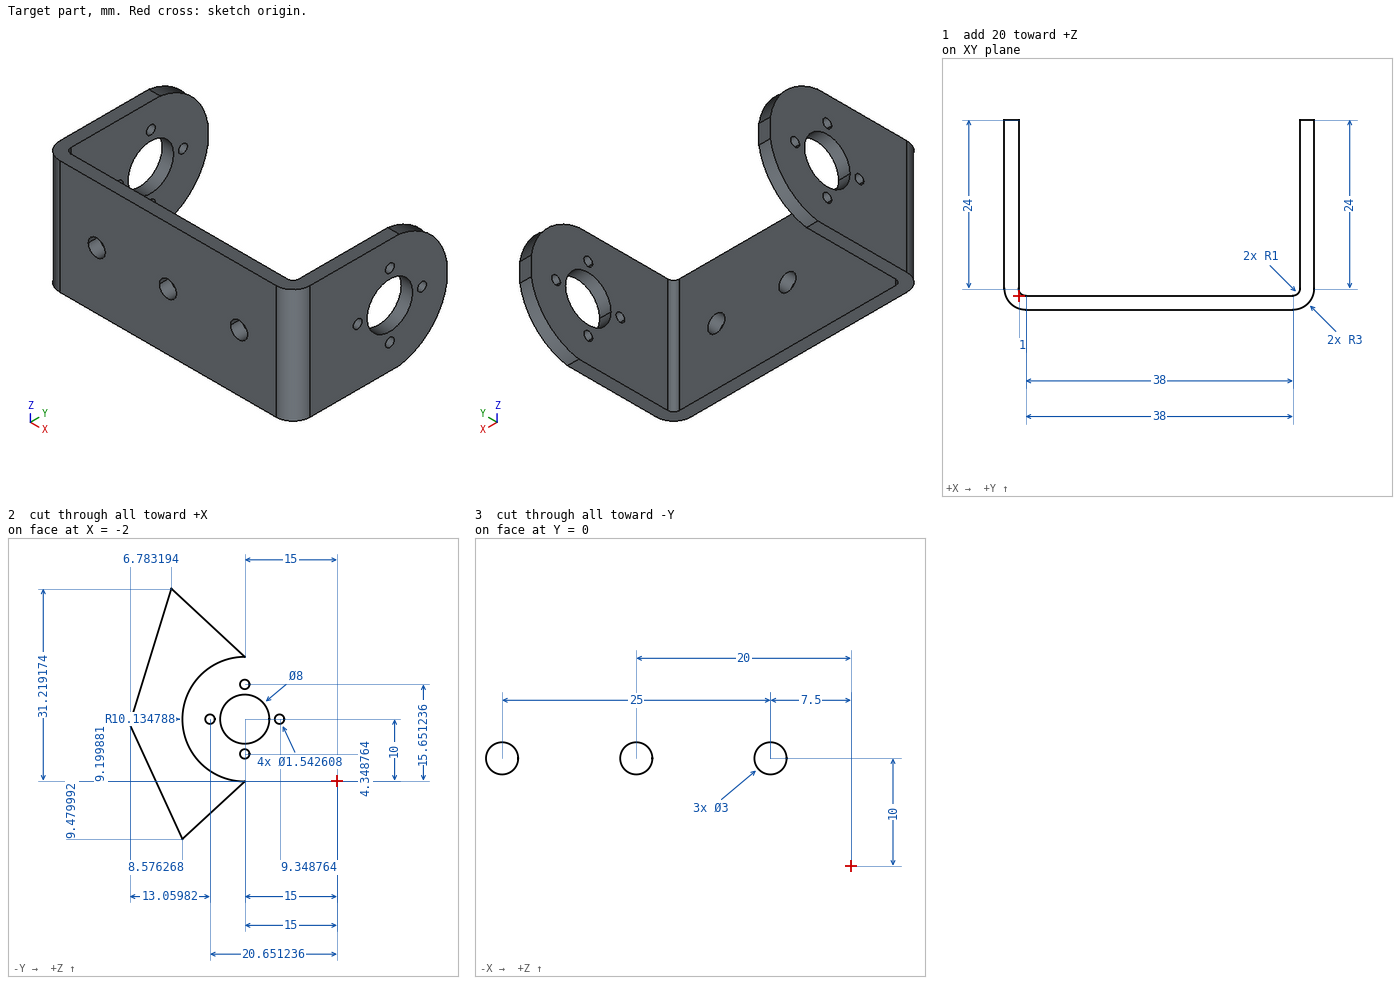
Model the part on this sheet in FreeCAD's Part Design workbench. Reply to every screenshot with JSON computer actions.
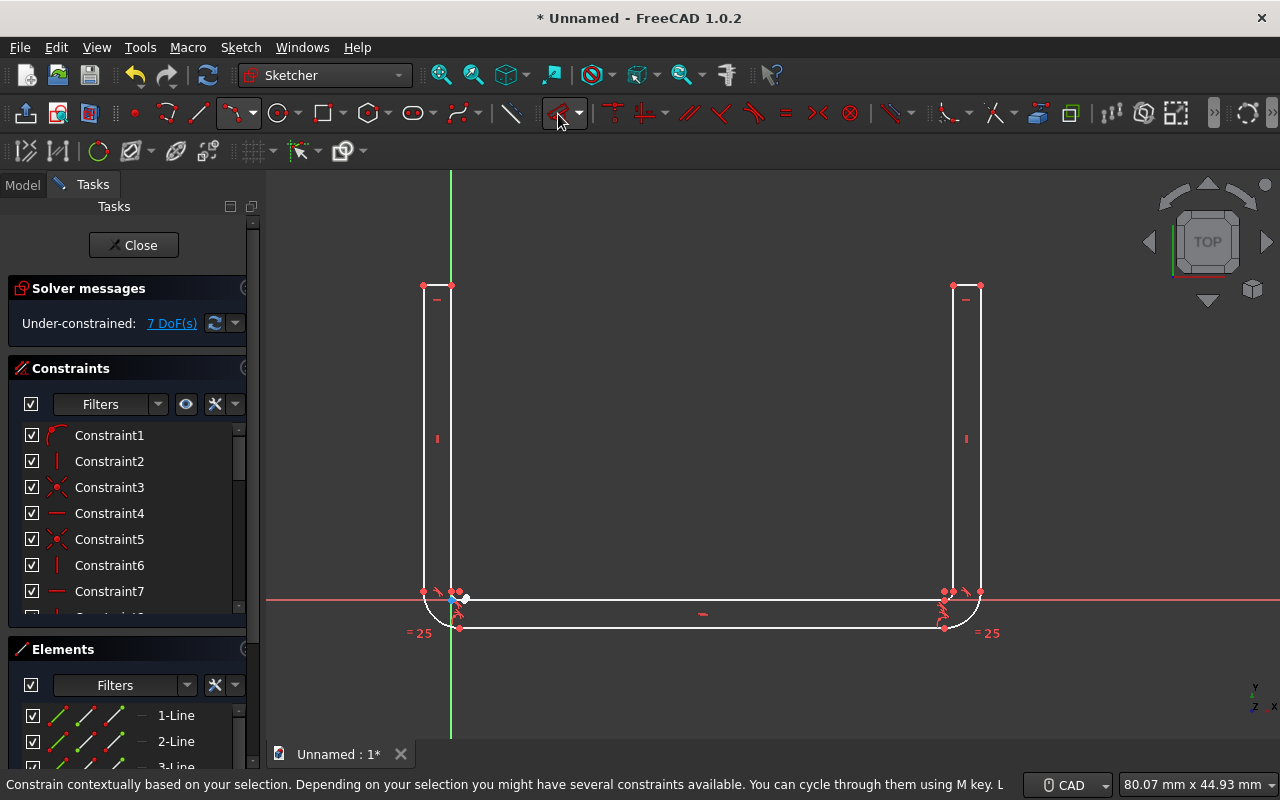
{"action": "left_click", "coordinate": [434, 617]}
{"action": "left_click", "coordinate": [411, 639]}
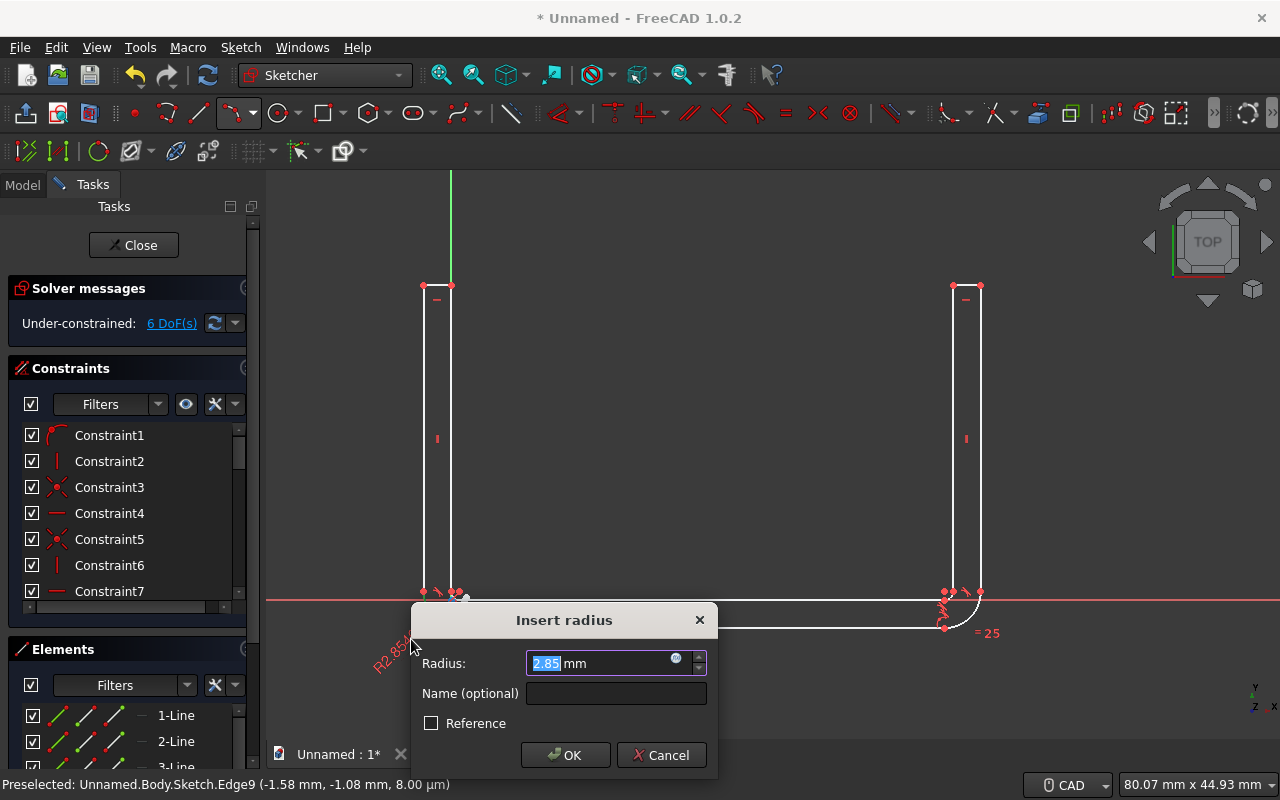
{"action": "type", "text": "3"}
{"action": "key", "text": "Return"}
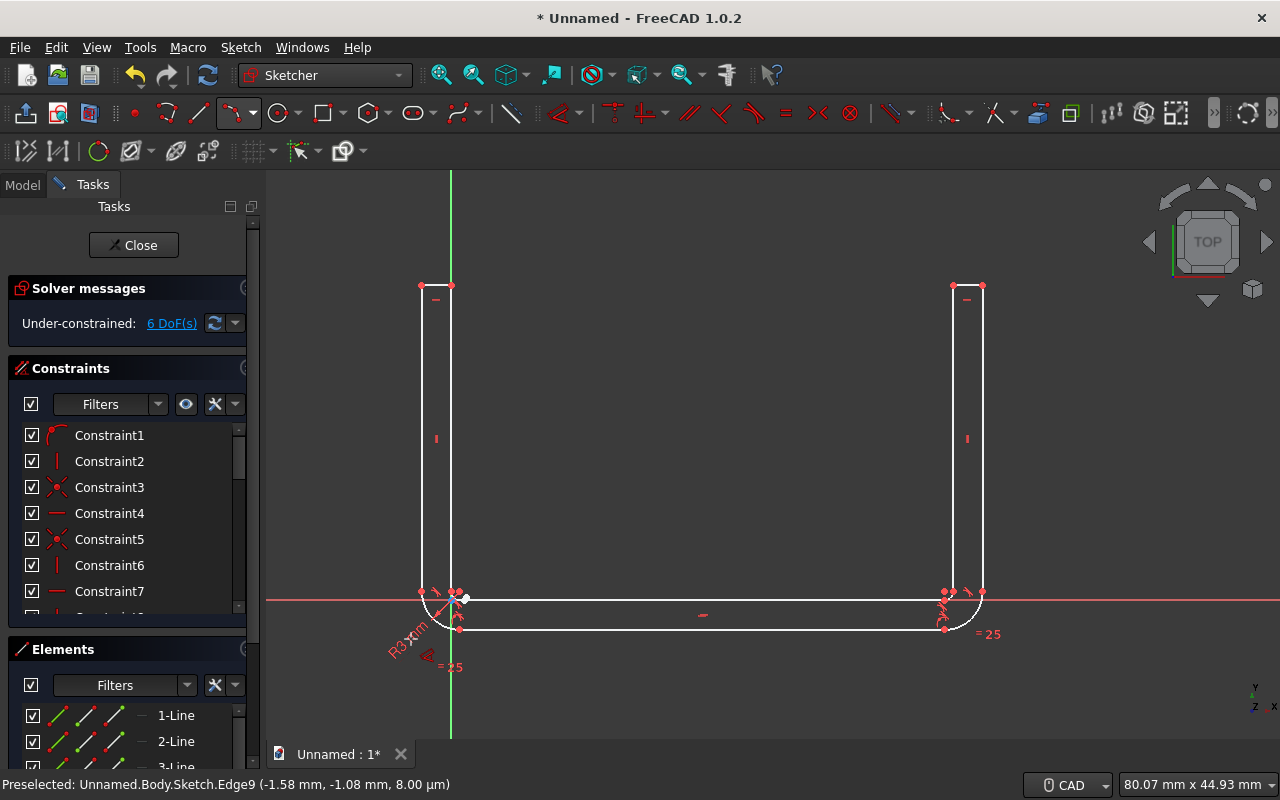
{"action": "scroll", "coordinate": [951, 598], "scroll_direction": "up", "scroll_amount": 6}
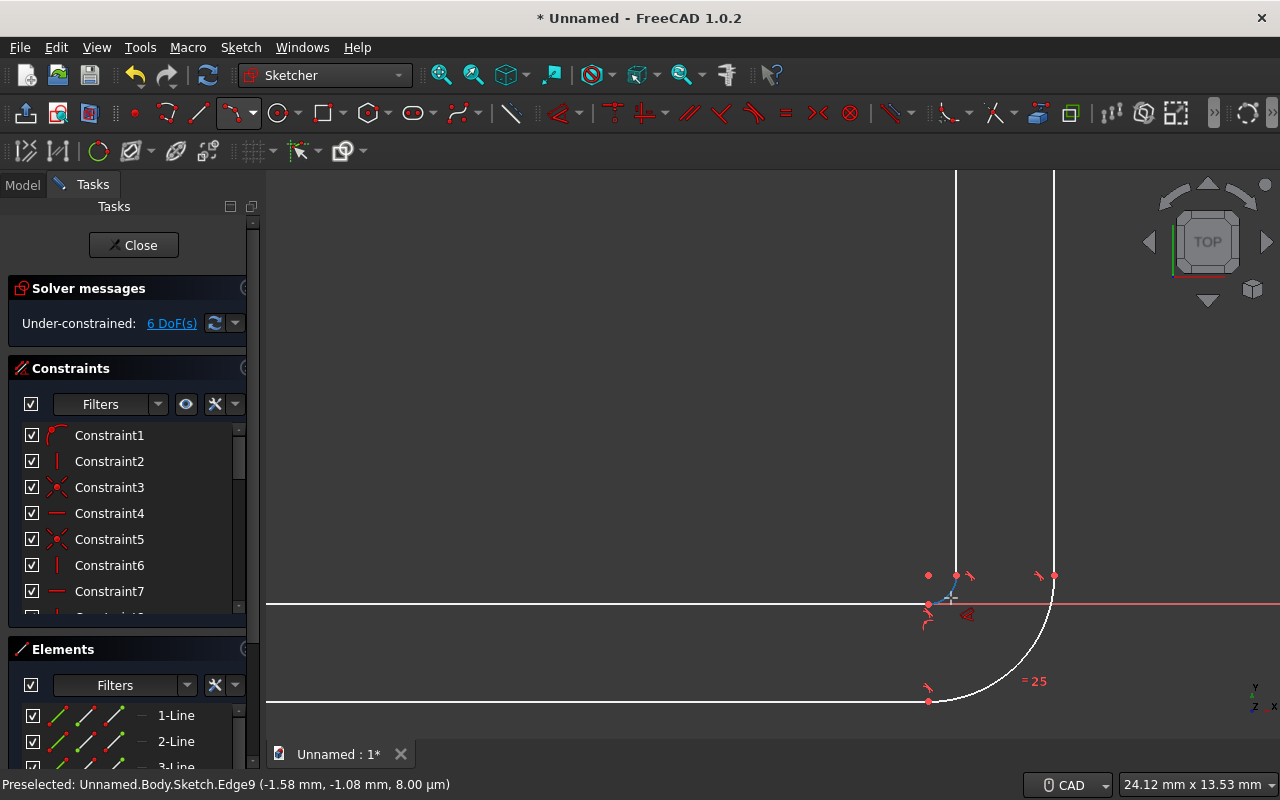
{"action": "left_click", "coordinate": [948, 596]}
{"action": "left_click", "coordinate": [971, 619]}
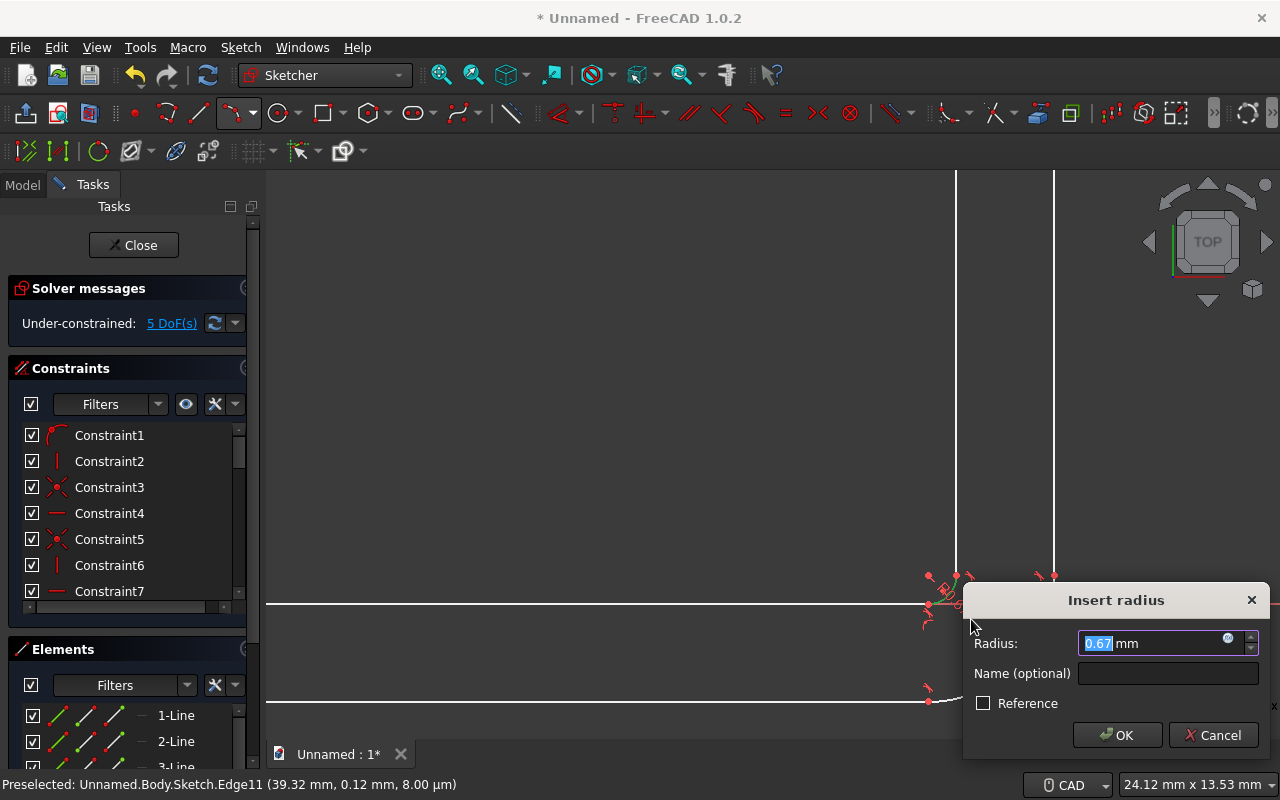
{"action": "type", "text": "1"}
{"action": "key", "text": "Return"}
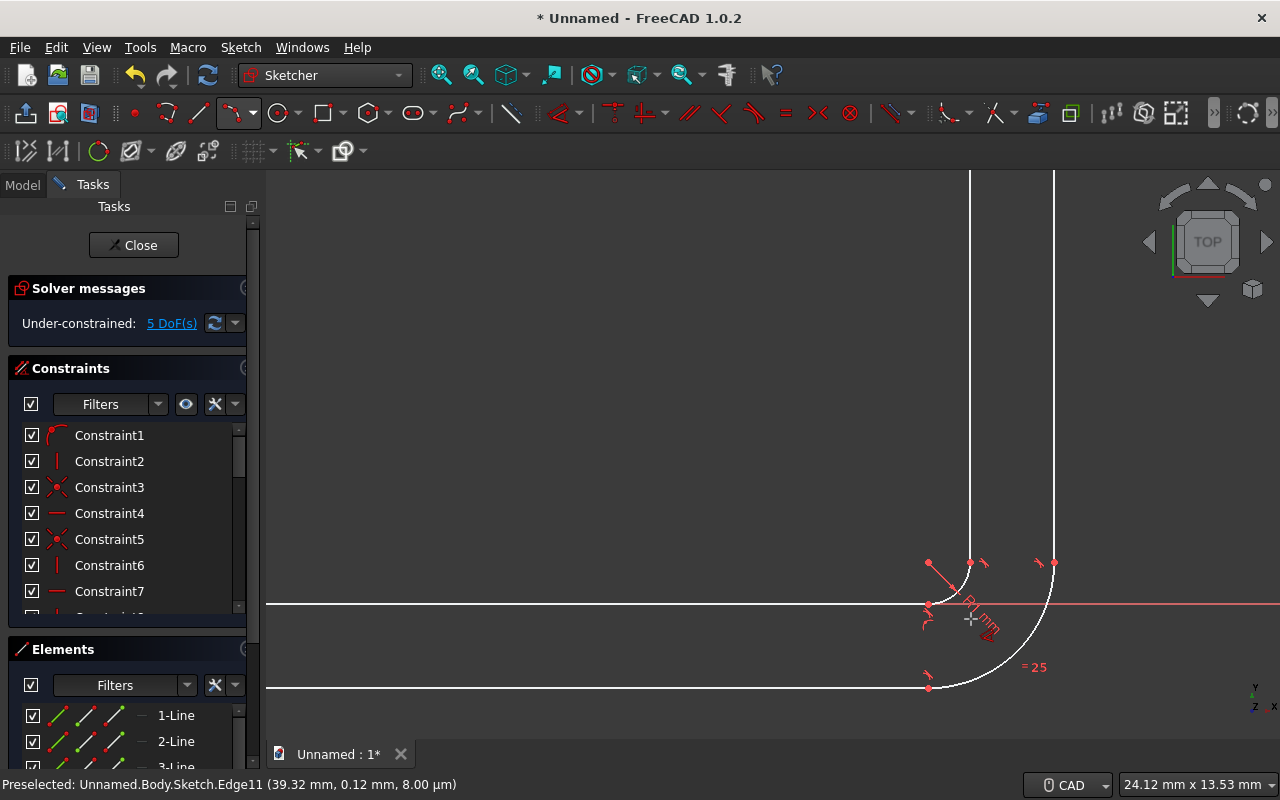
{"action": "scroll", "coordinate": [951, 598], "scroll_direction": "down", "scroll_amount": 6}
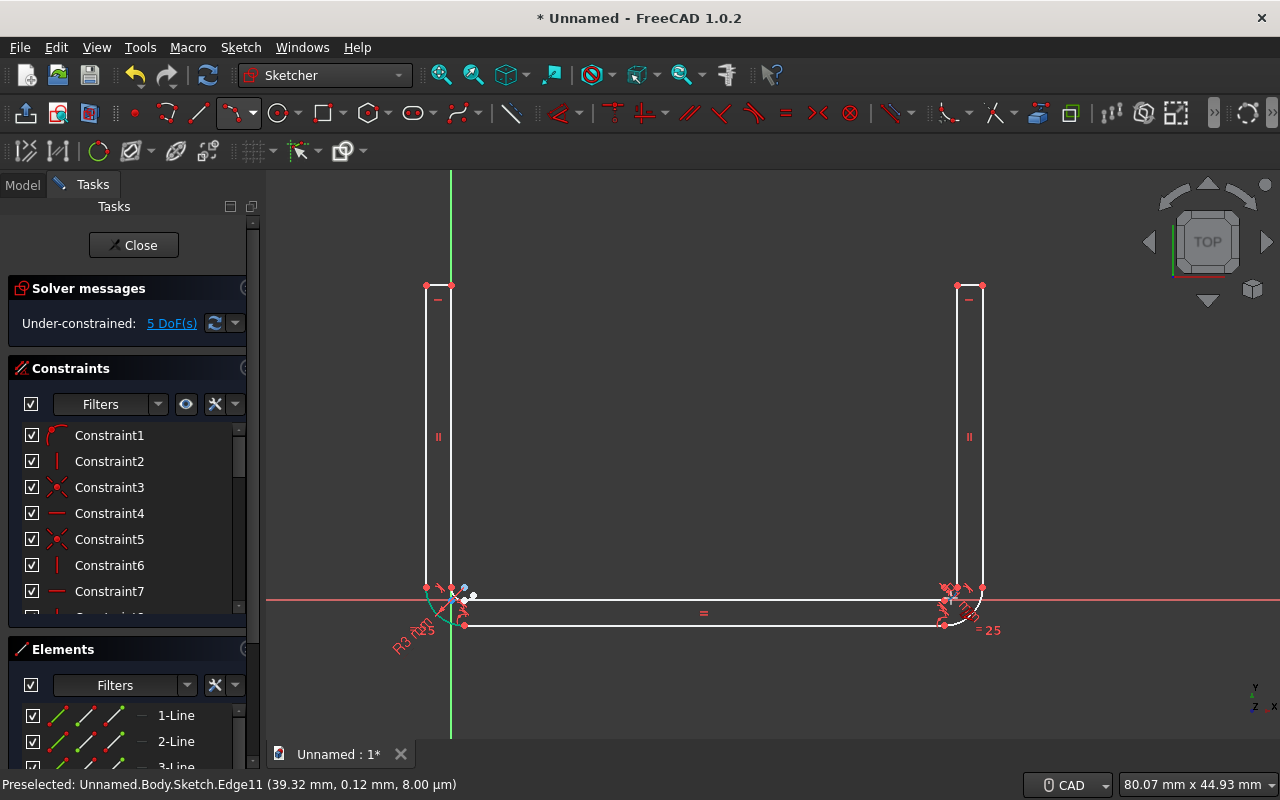
{"action": "left_click", "coordinate": [451, 497]}
{"action": "left_click", "coordinate": [485, 436]}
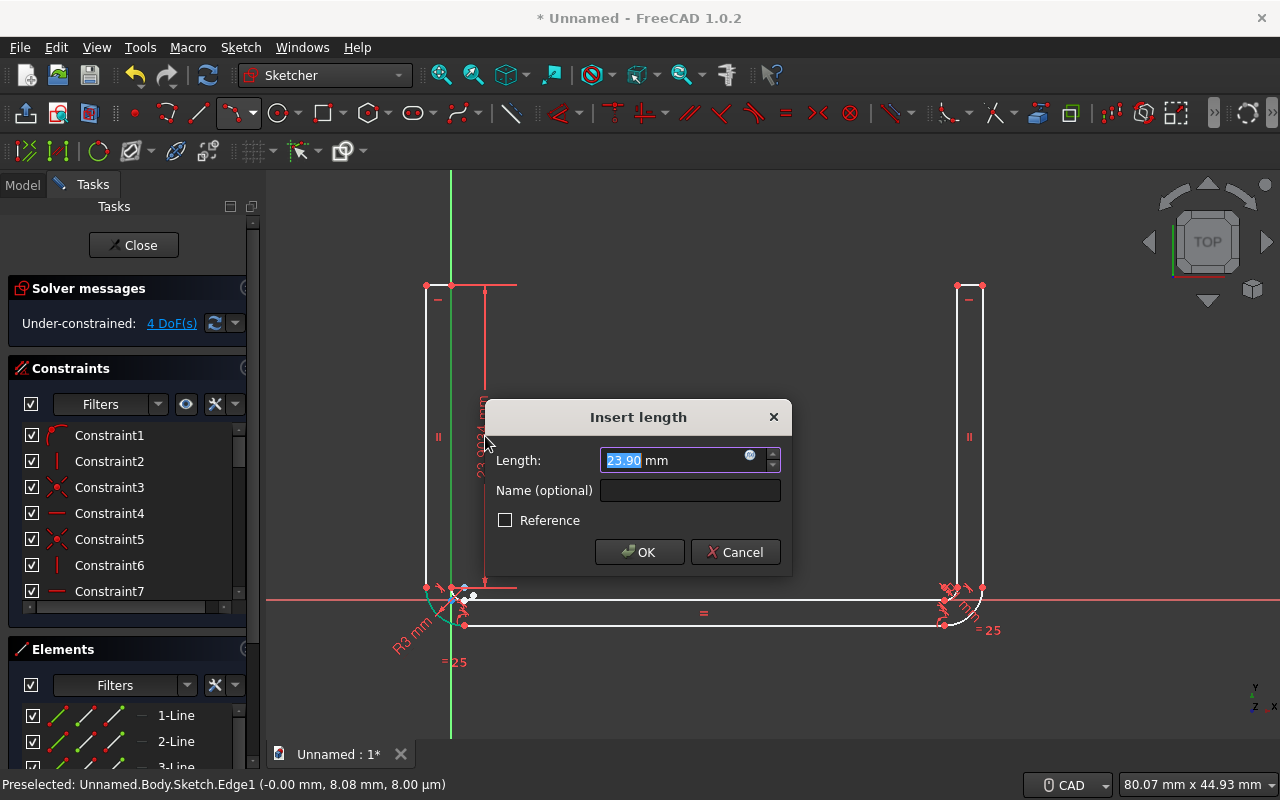
{"action": "type", "text": "24"}
{"action": "key", "text": "Return"}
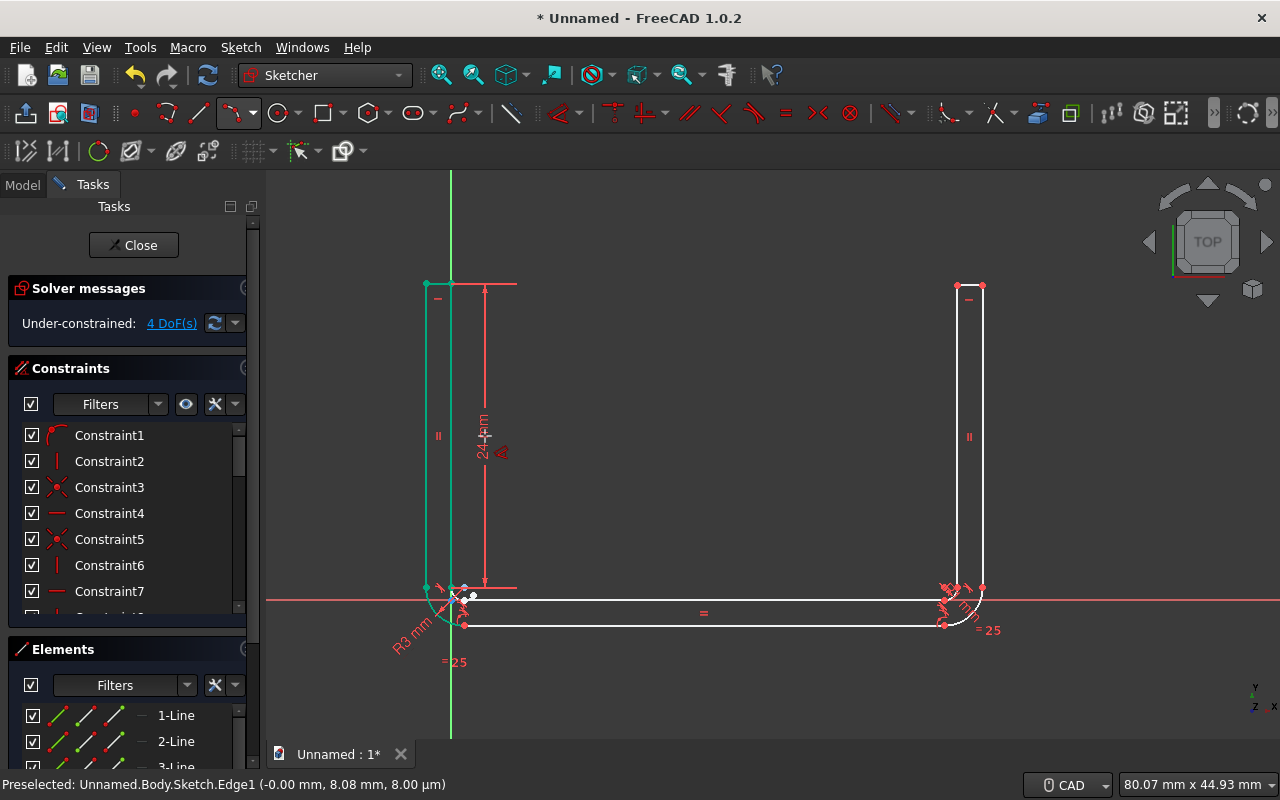
{"action": "left_click", "coordinate": [608, 626]}
{"action": "left_click", "coordinate": [704, 660]}